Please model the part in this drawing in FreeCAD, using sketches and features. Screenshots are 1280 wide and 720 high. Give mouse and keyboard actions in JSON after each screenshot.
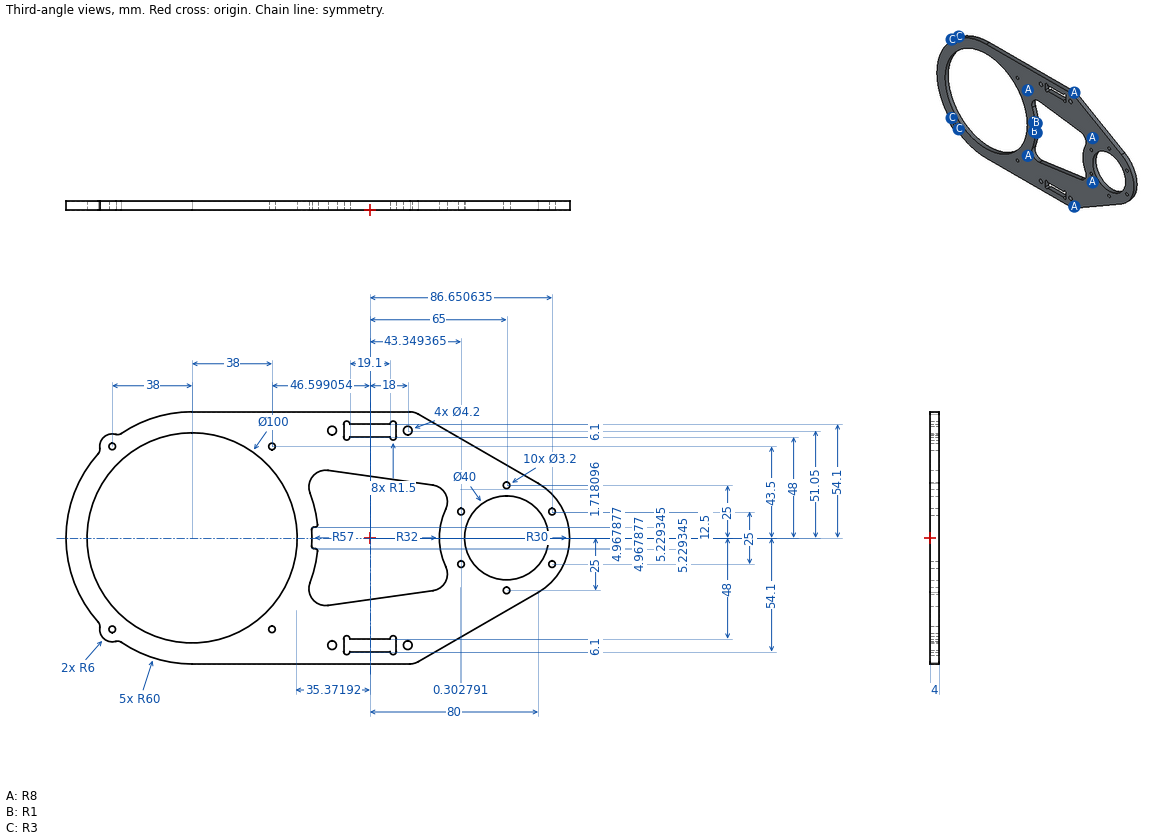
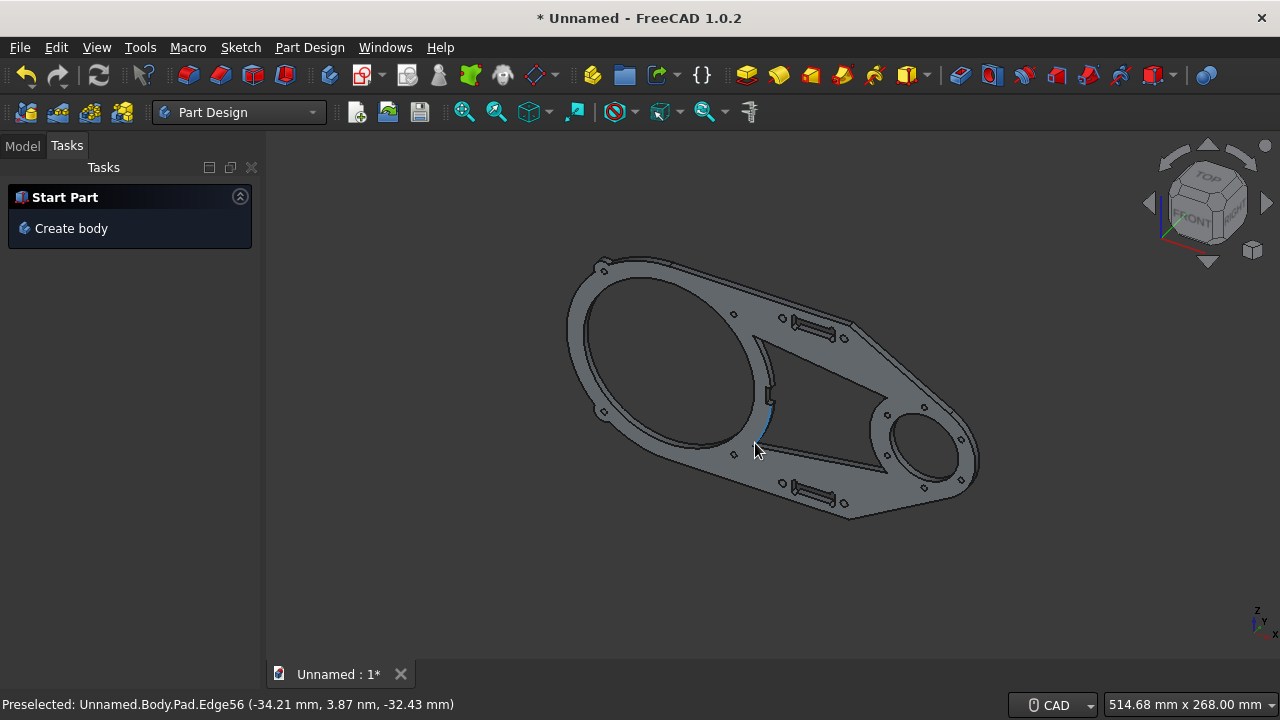
{"action": "key", "text": "0"}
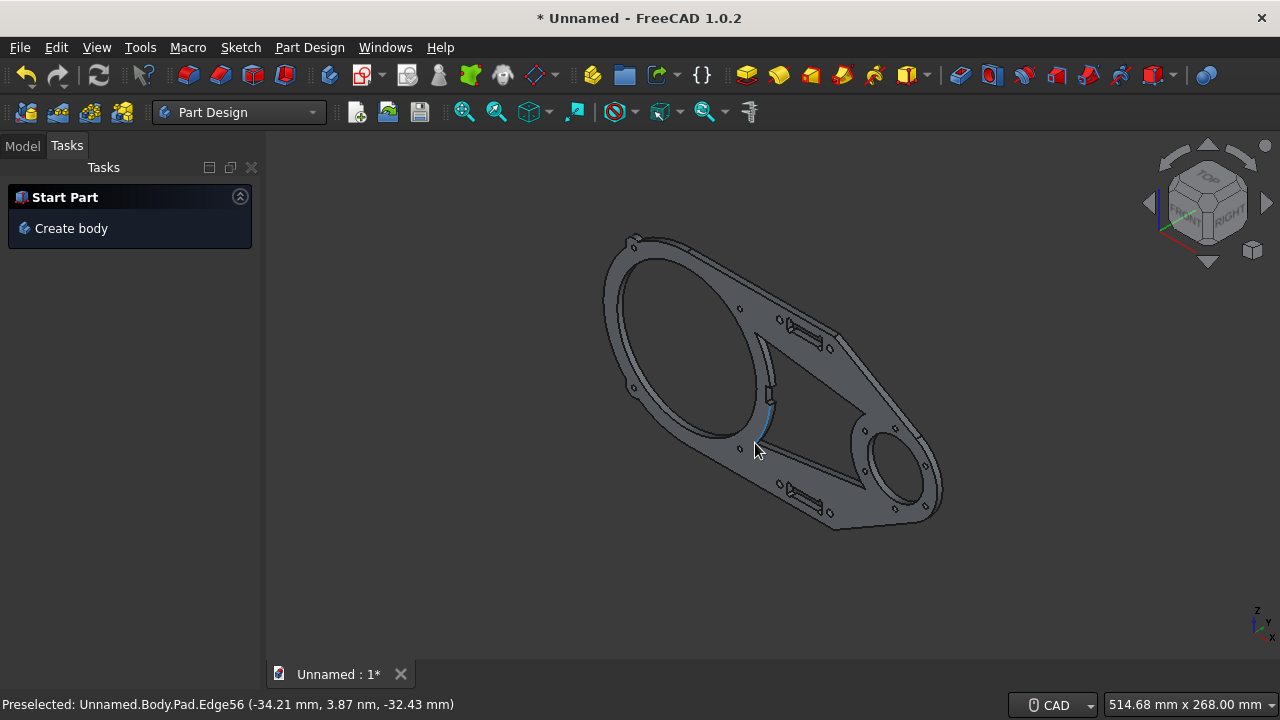
{"action": "scroll", "coordinate": [758, 441], "scroll_direction": "up", "scroll_amount": 9}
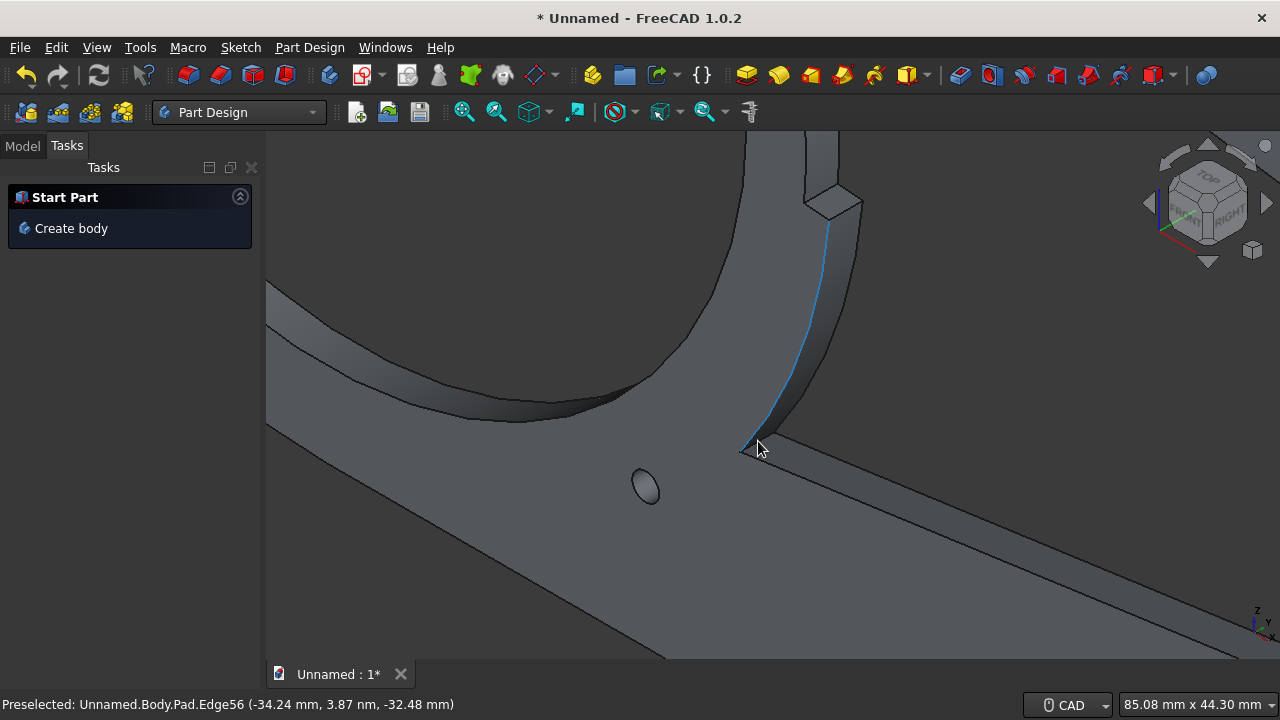
{"action": "left_click", "coordinate": [466, 112]}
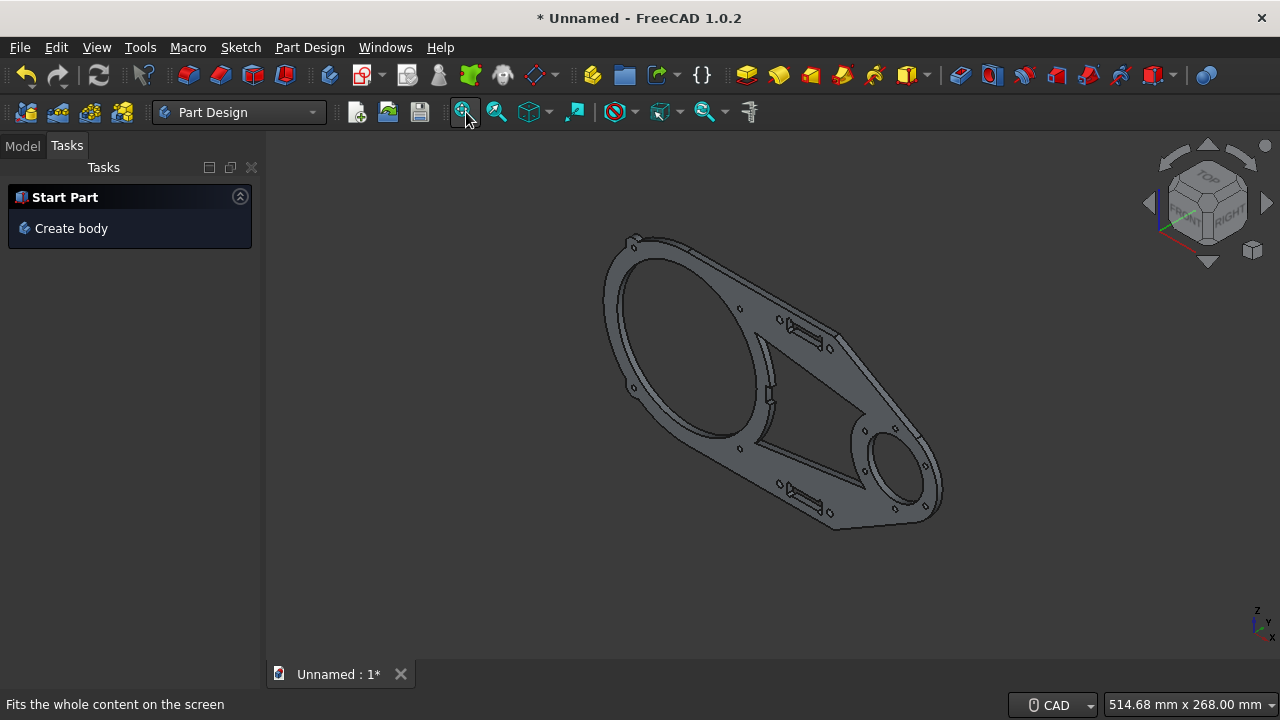
{"action": "key", "text": "2"}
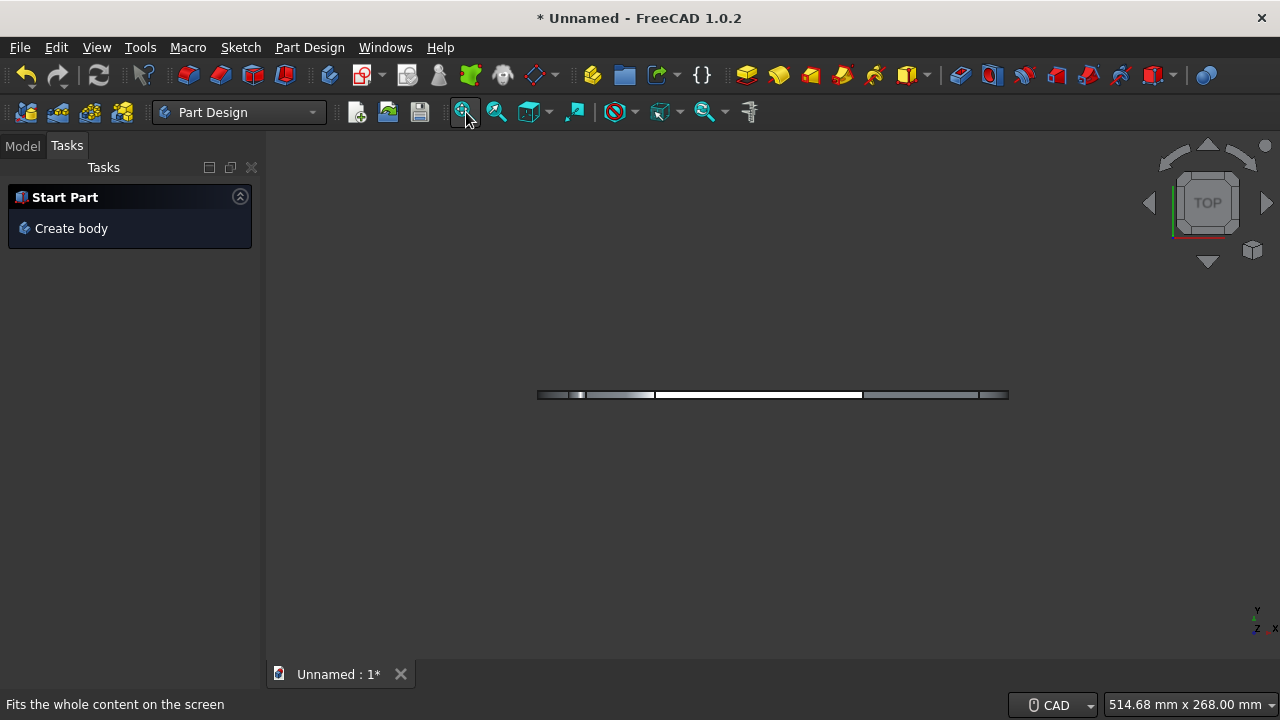
{"action": "scroll", "coordinate": [752, 394], "scroll_direction": "up", "scroll_amount": 9}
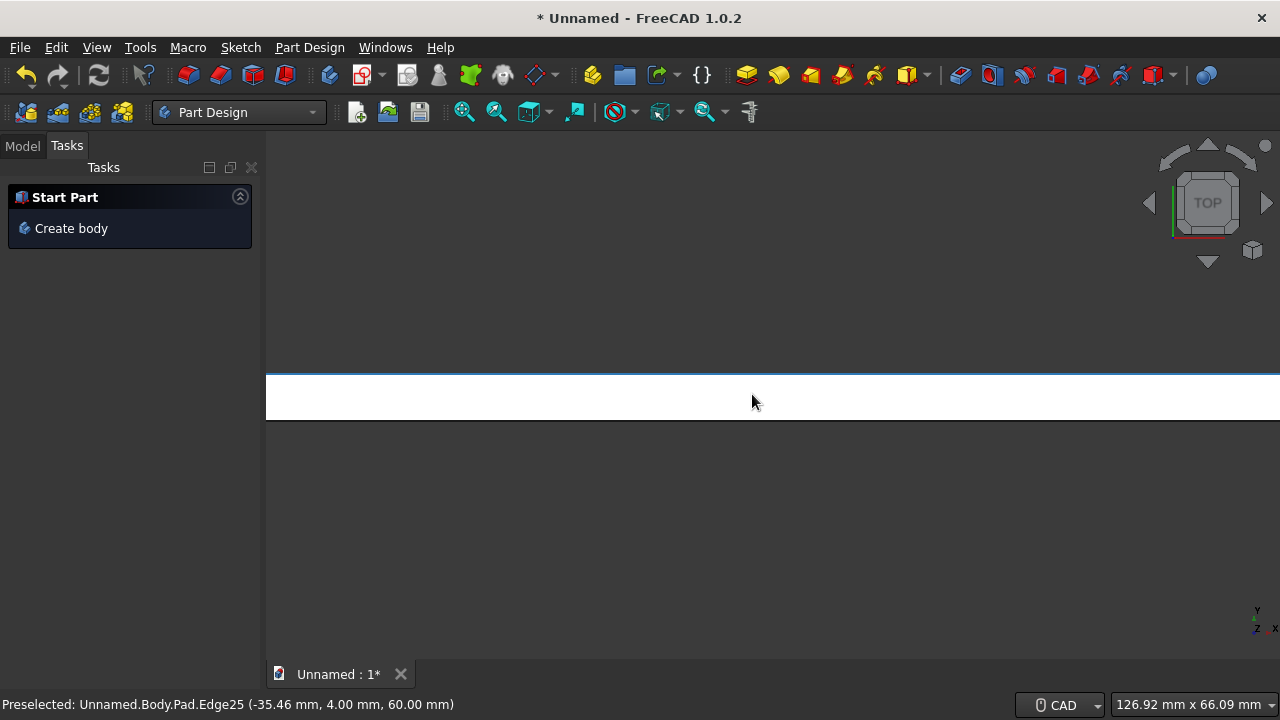
{"action": "left_click", "coordinate": [466, 112]}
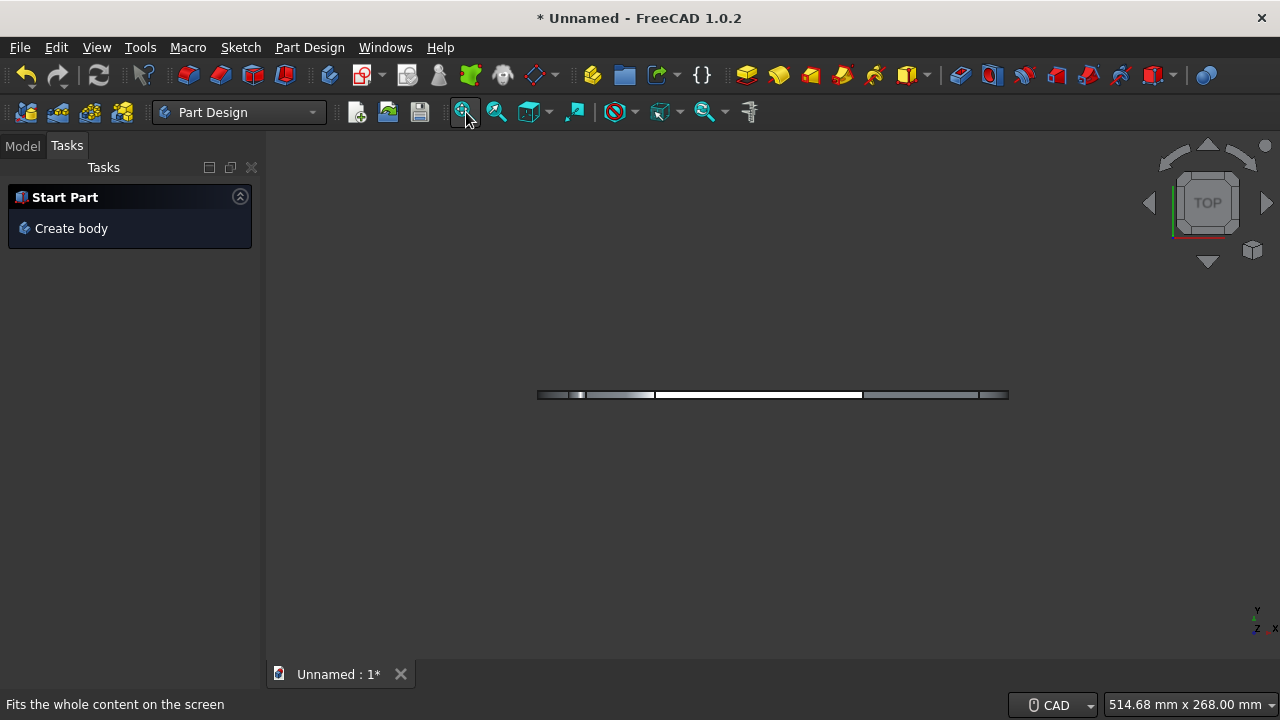
{"action": "key", "text": "1"}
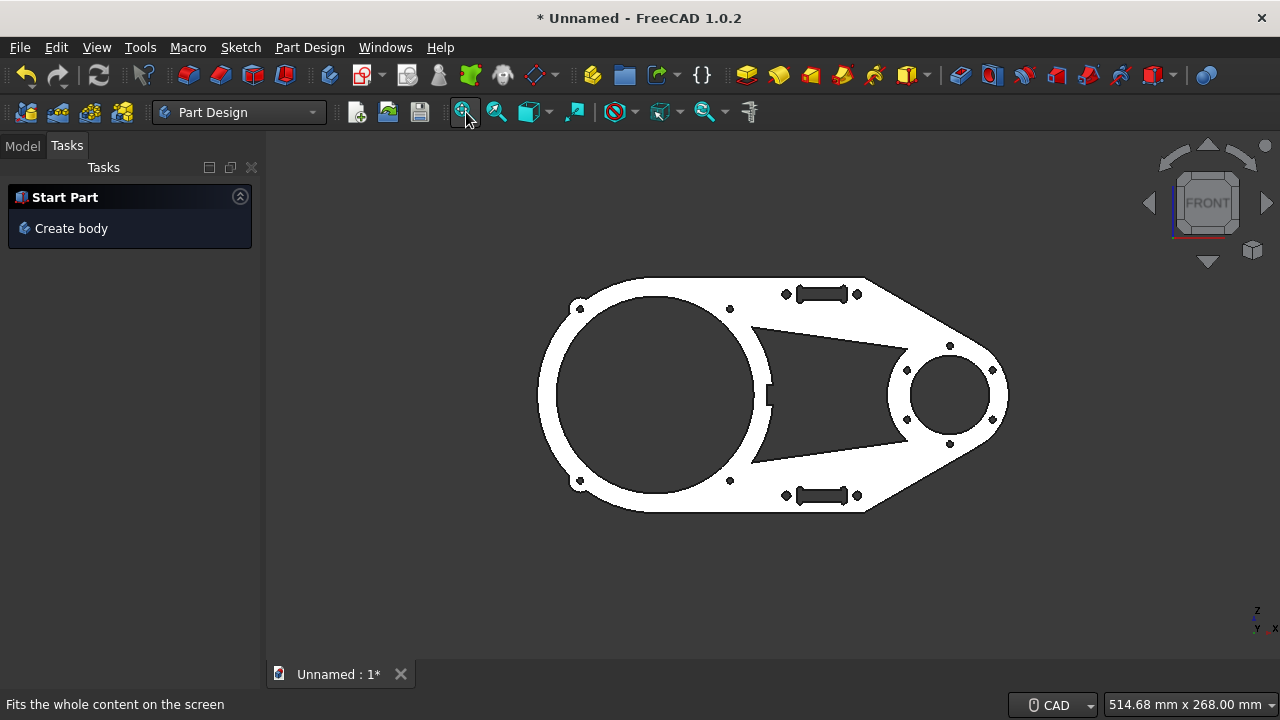
{"action": "scroll", "coordinate": [752, 462], "scroll_direction": "up", "scroll_amount": 9}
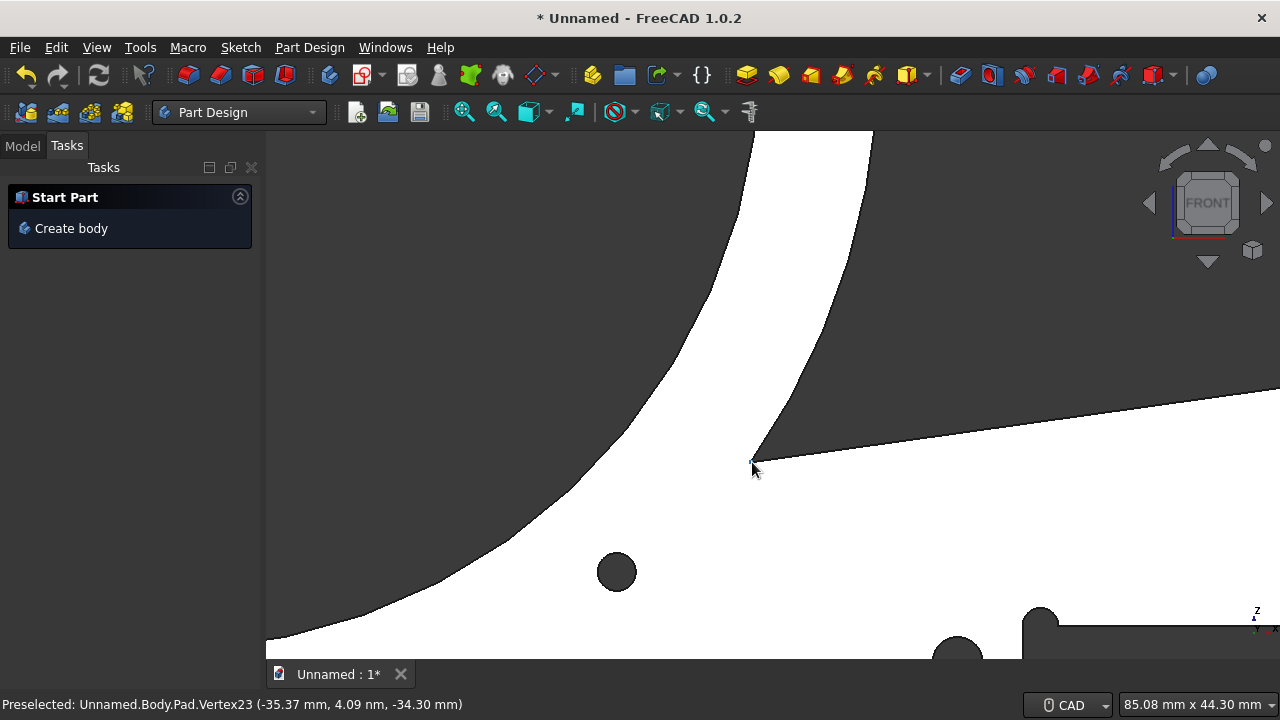
{"action": "left_click", "coordinate": [466, 112]}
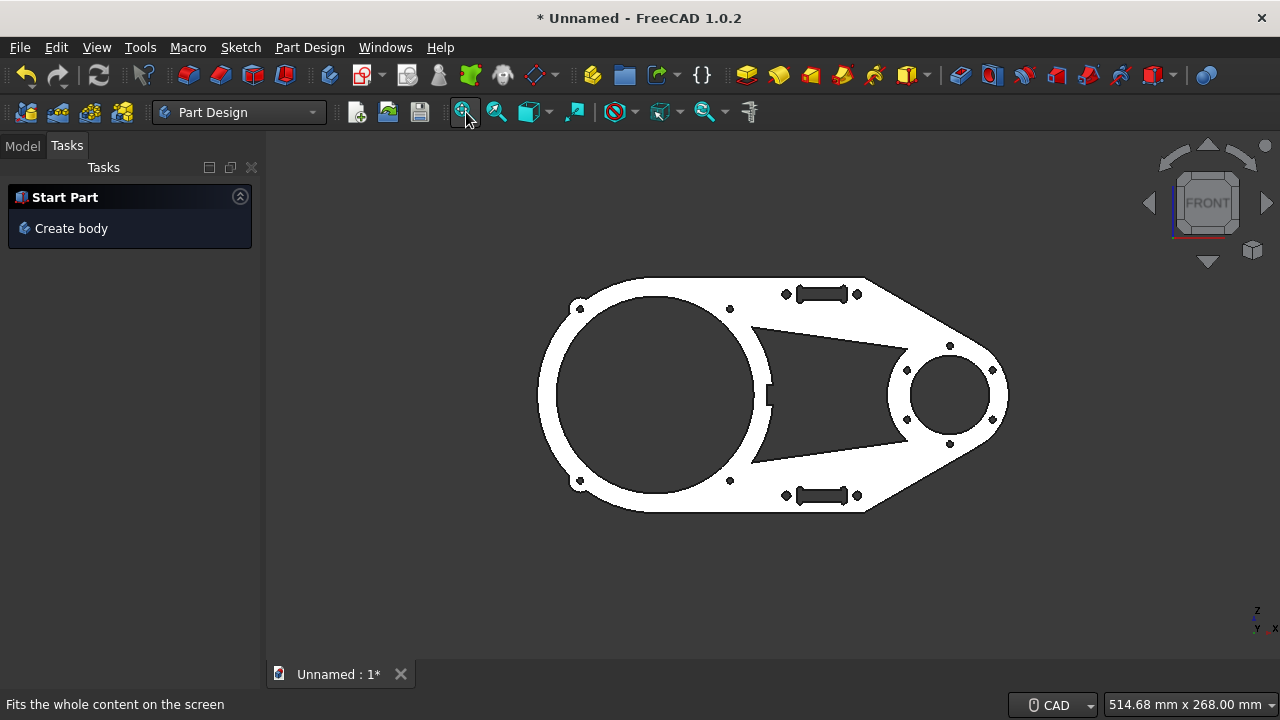
{"action": "key", "text": "3"}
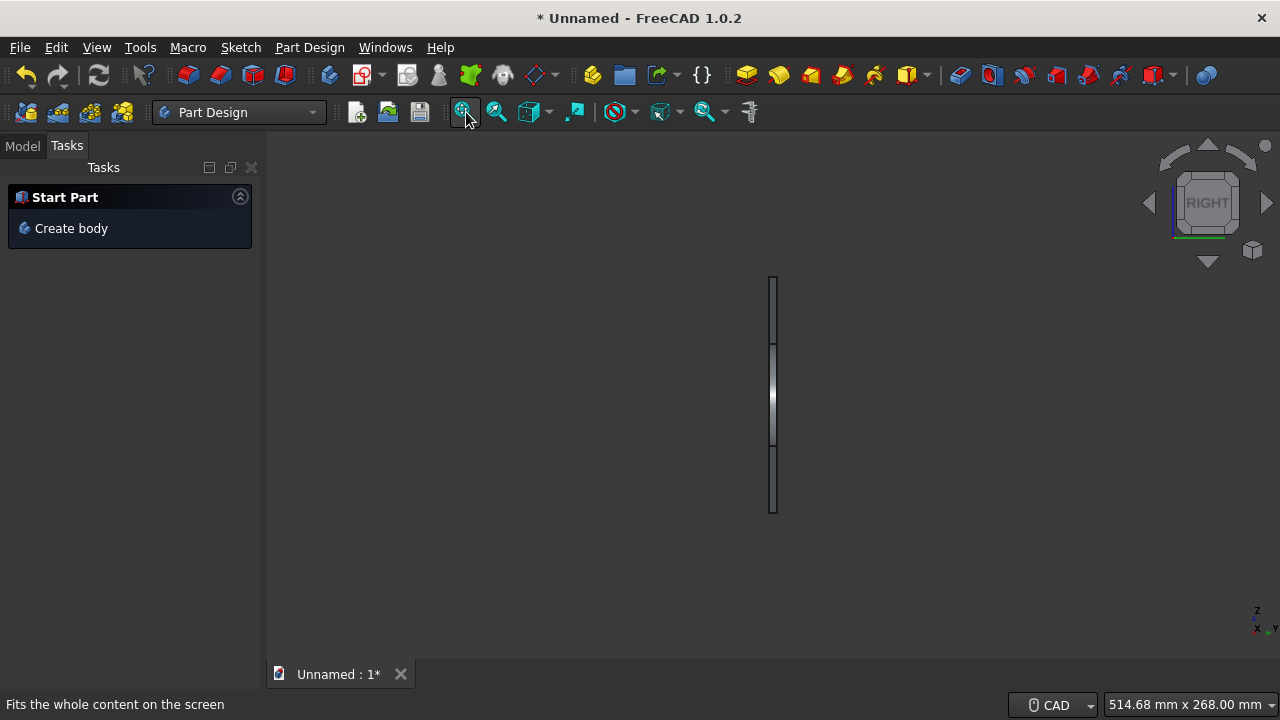
{"action": "left_click", "coordinate": [466, 112]}